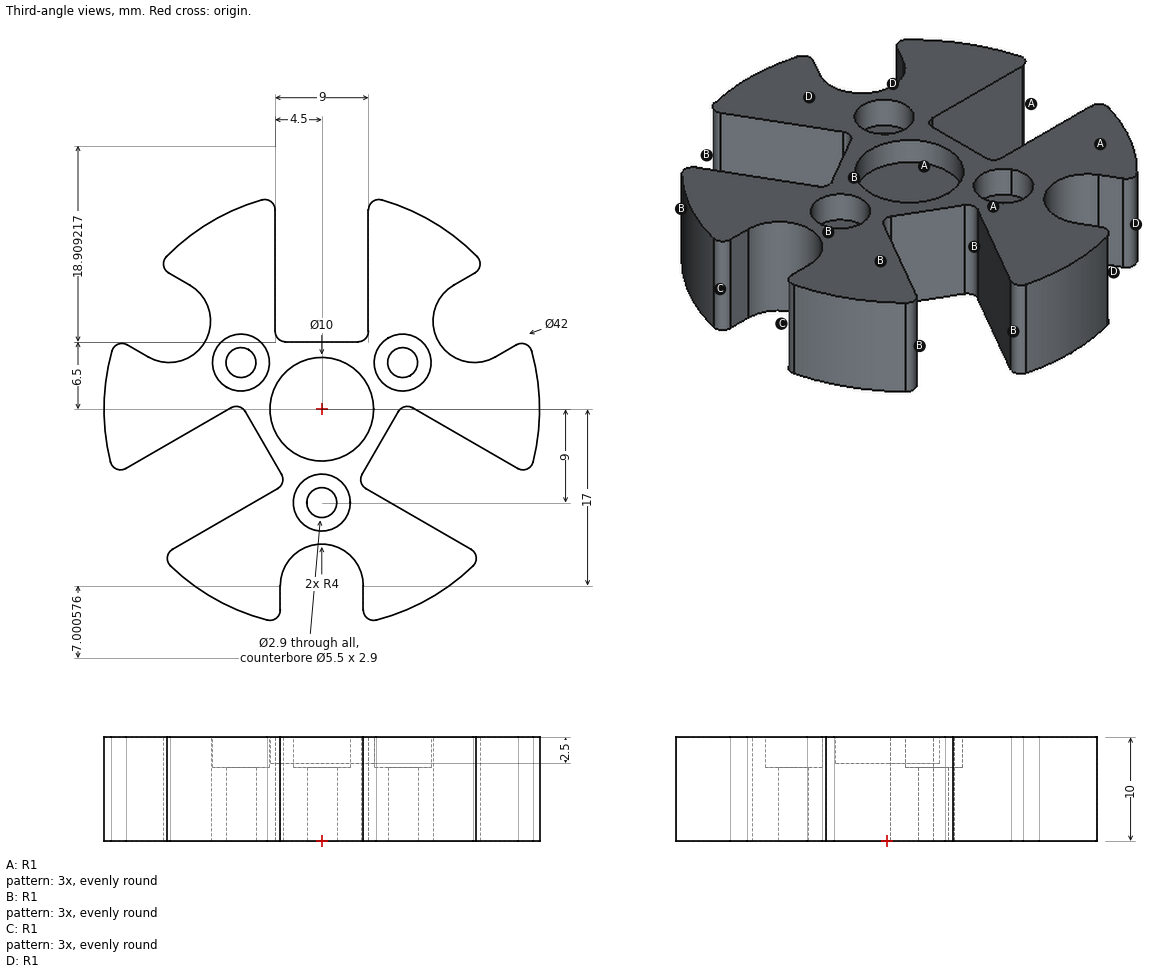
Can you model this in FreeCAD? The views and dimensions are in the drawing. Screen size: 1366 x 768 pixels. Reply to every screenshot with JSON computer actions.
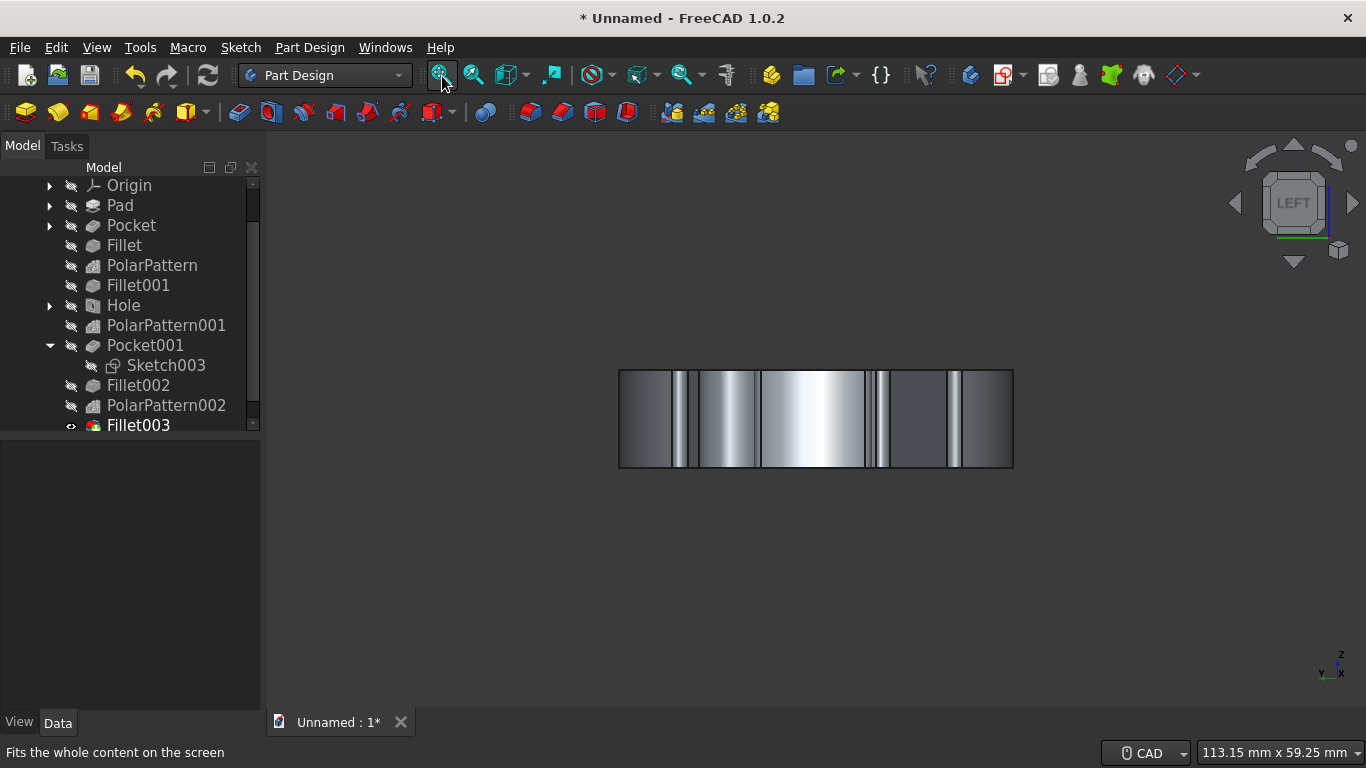
{"action": "key", "text": "0"}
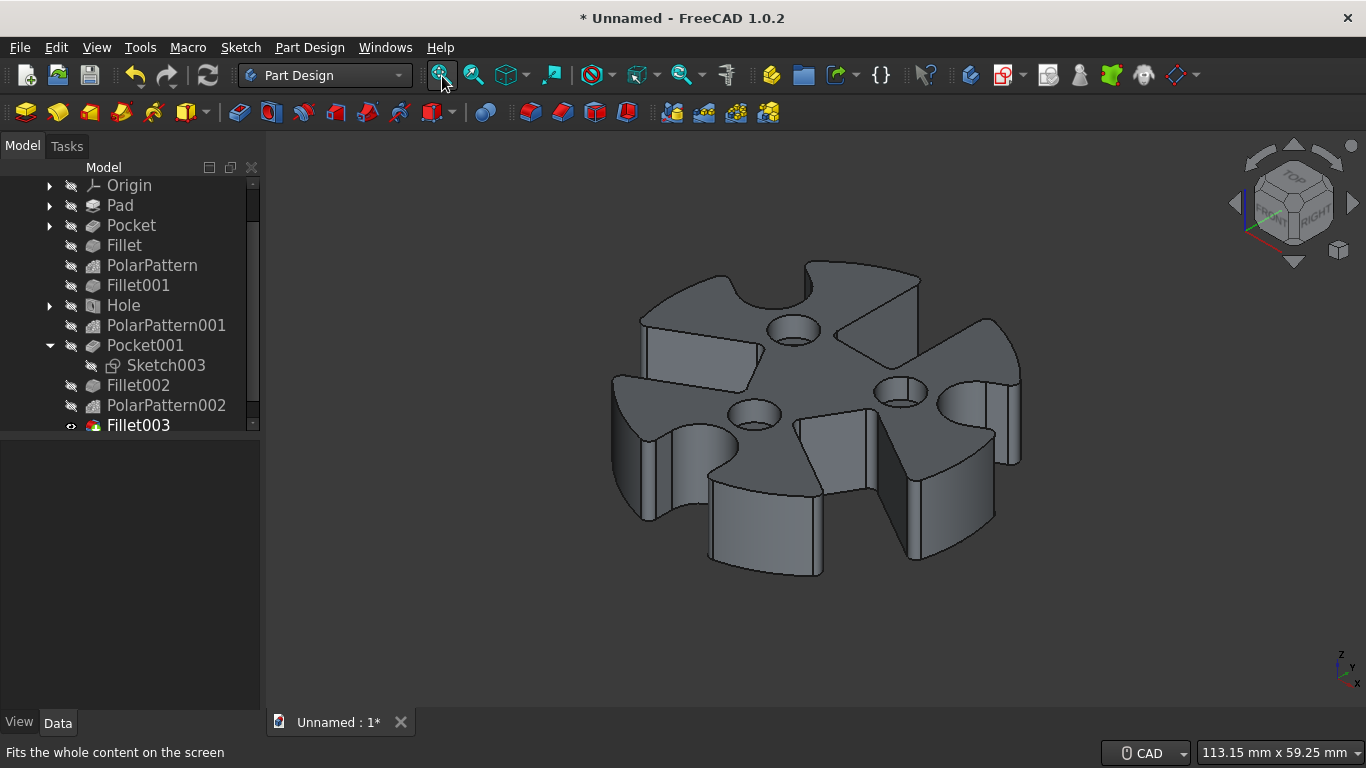
{"action": "left_click", "coordinate": [816, 378]}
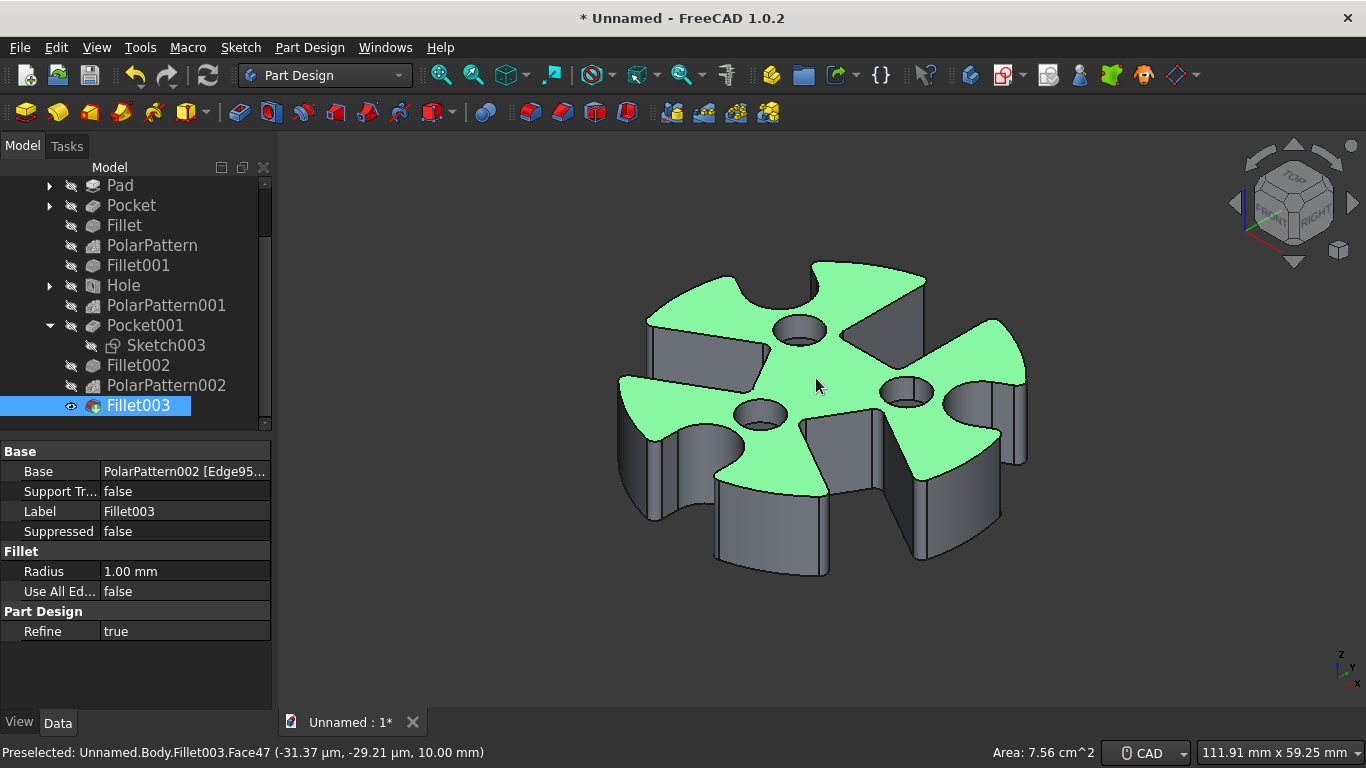
{"action": "left_click", "coordinate": [1004, 76]}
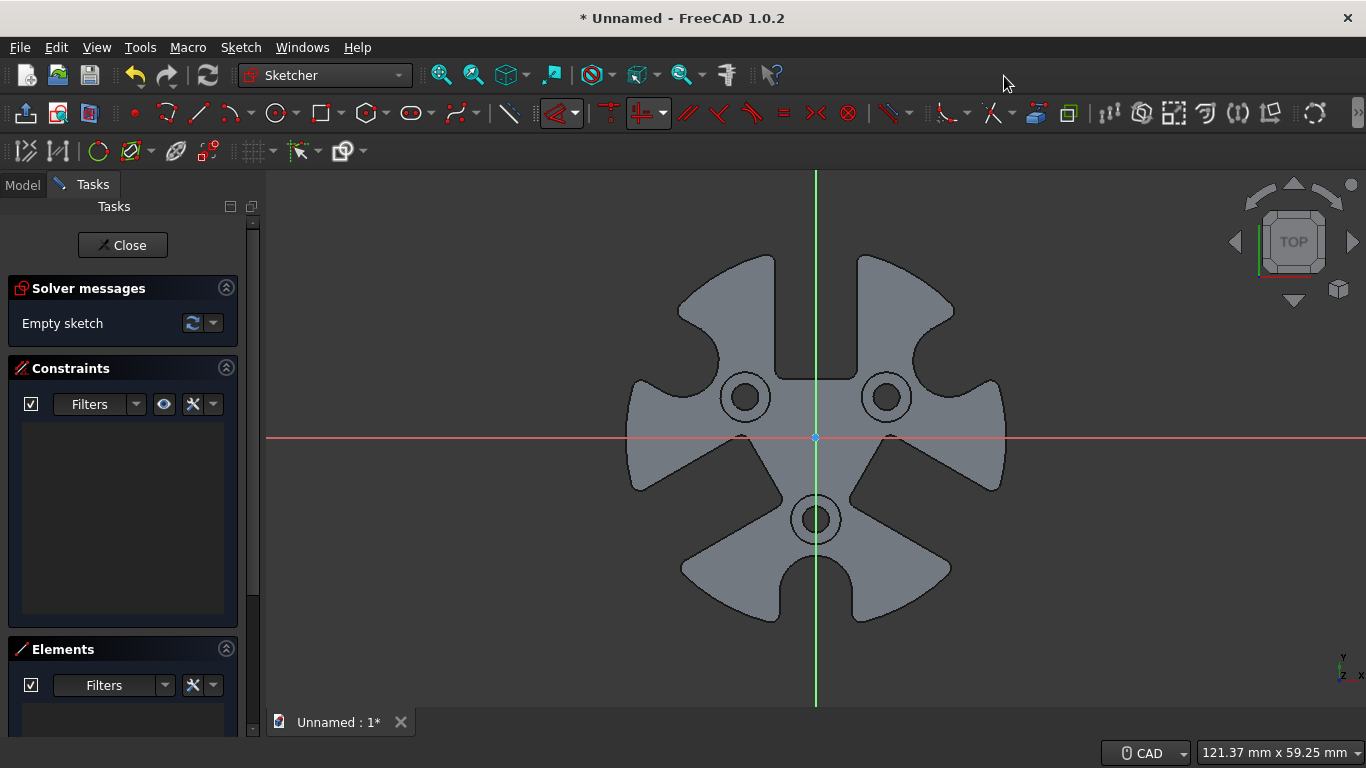
{"action": "scroll", "coordinate": [838, 438], "scroll_direction": "up", "scroll_amount": 7}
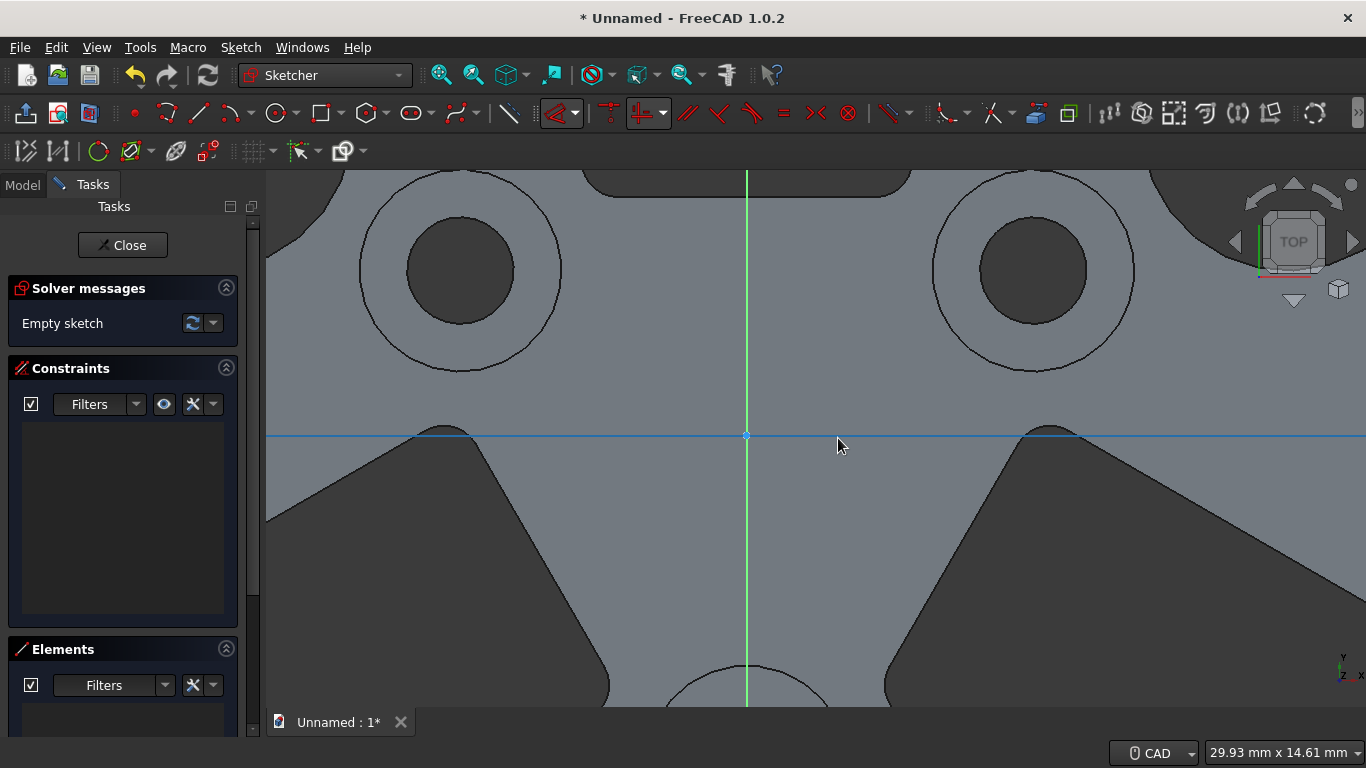
{"action": "left_click", "coordinate": [276, 114]}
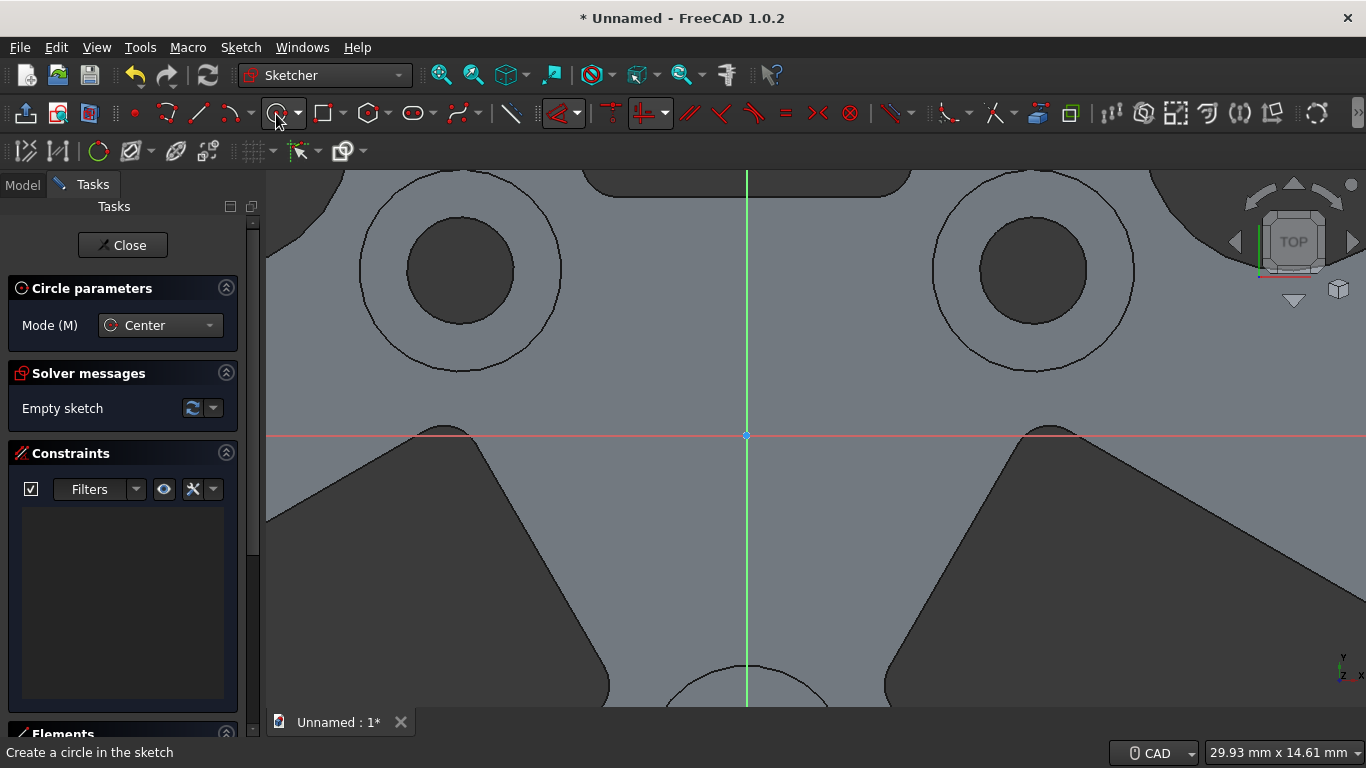
{"action": "left_click", "coordinate": [747, 436]}
{"action": "left_click", "coordinate": [877, 306]}
{"action": "key", "text": "Escape"}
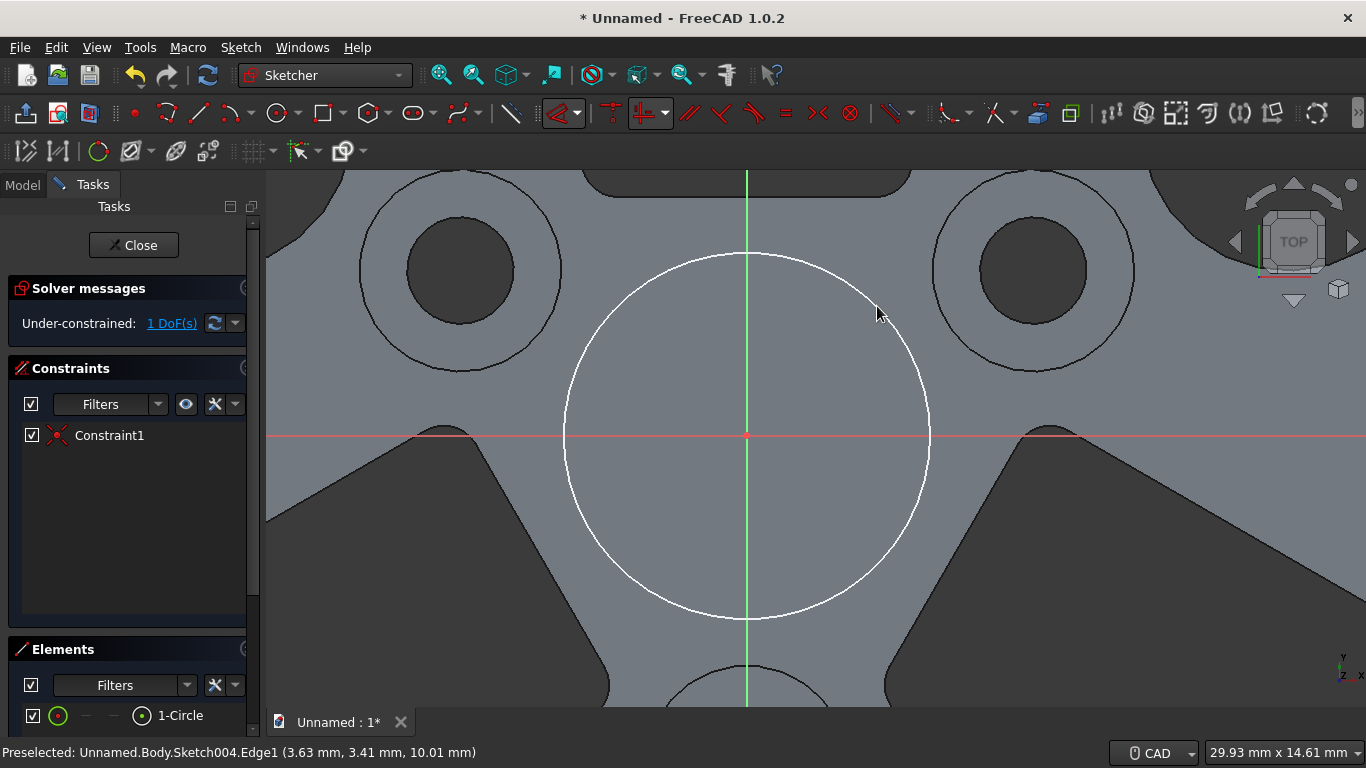
{"action": "left_click", "coordinate": [876, 306]}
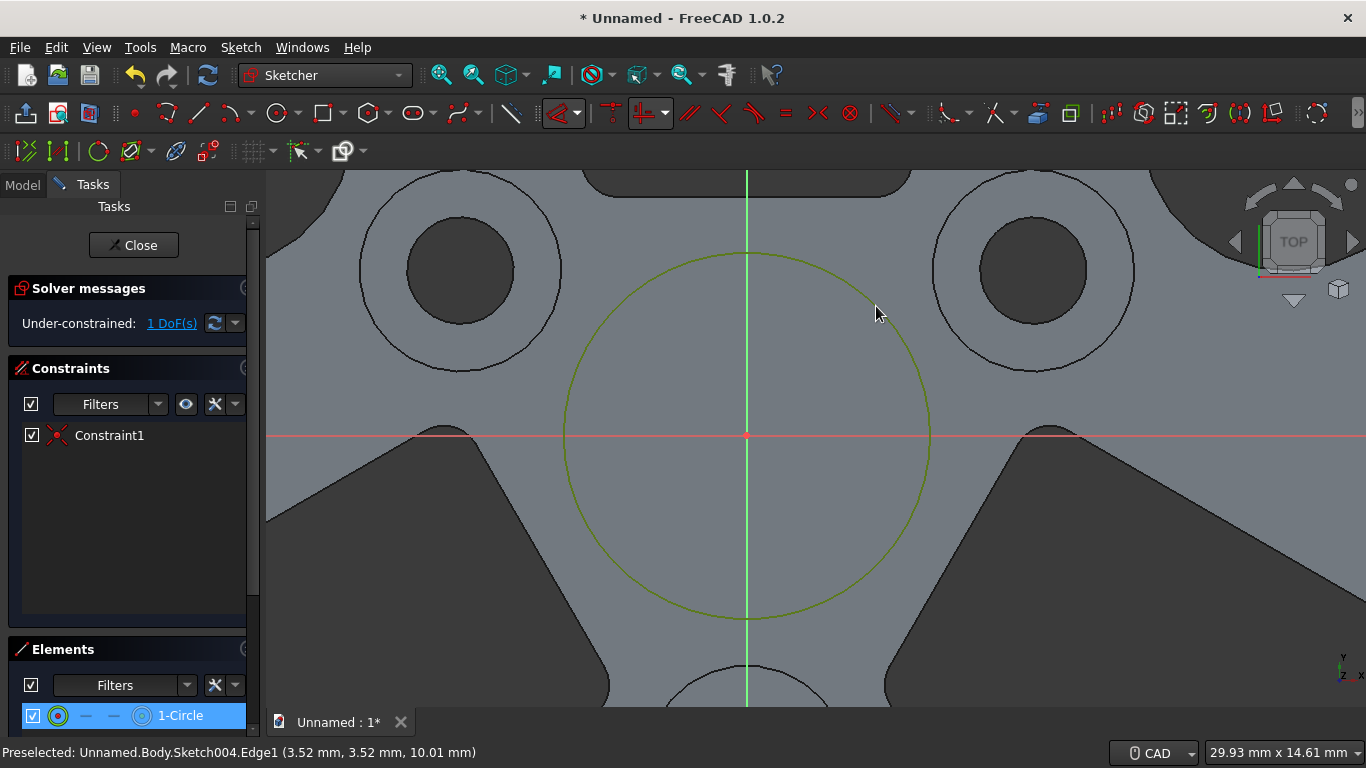
{"action": "key", "text": "k o"}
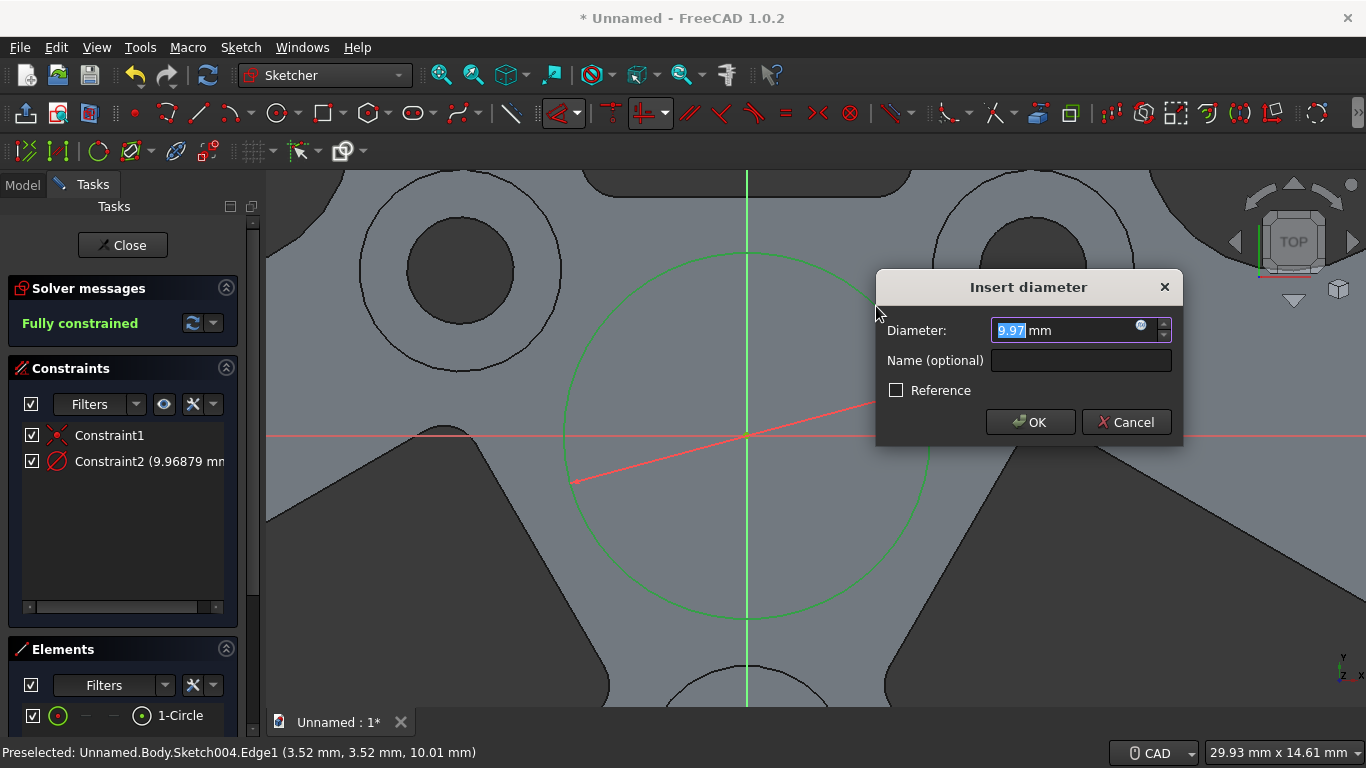
{"action": "type", "text": "10"}
{"action": "key", "text": "Return"}